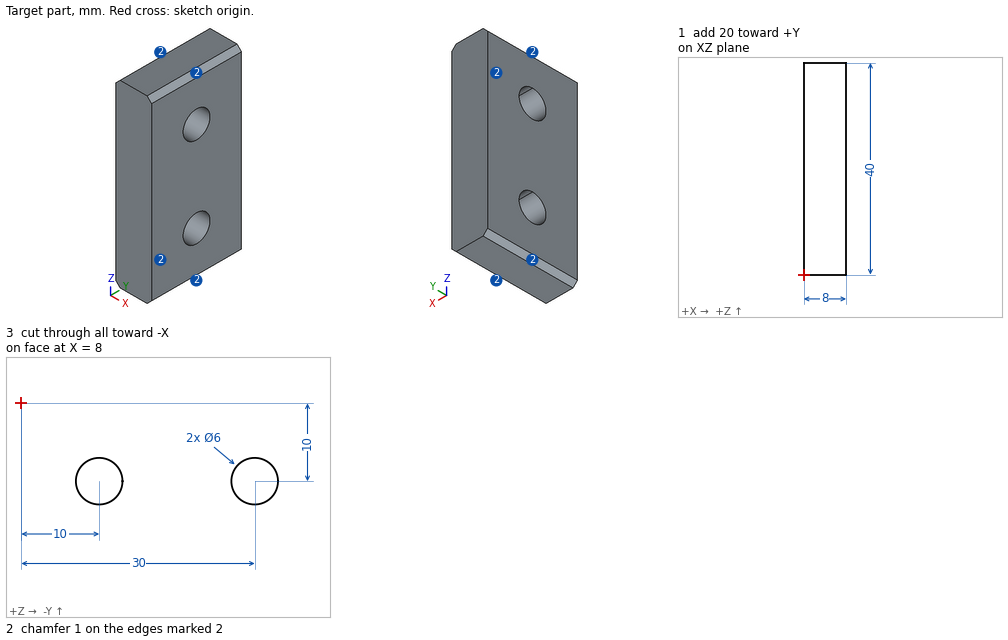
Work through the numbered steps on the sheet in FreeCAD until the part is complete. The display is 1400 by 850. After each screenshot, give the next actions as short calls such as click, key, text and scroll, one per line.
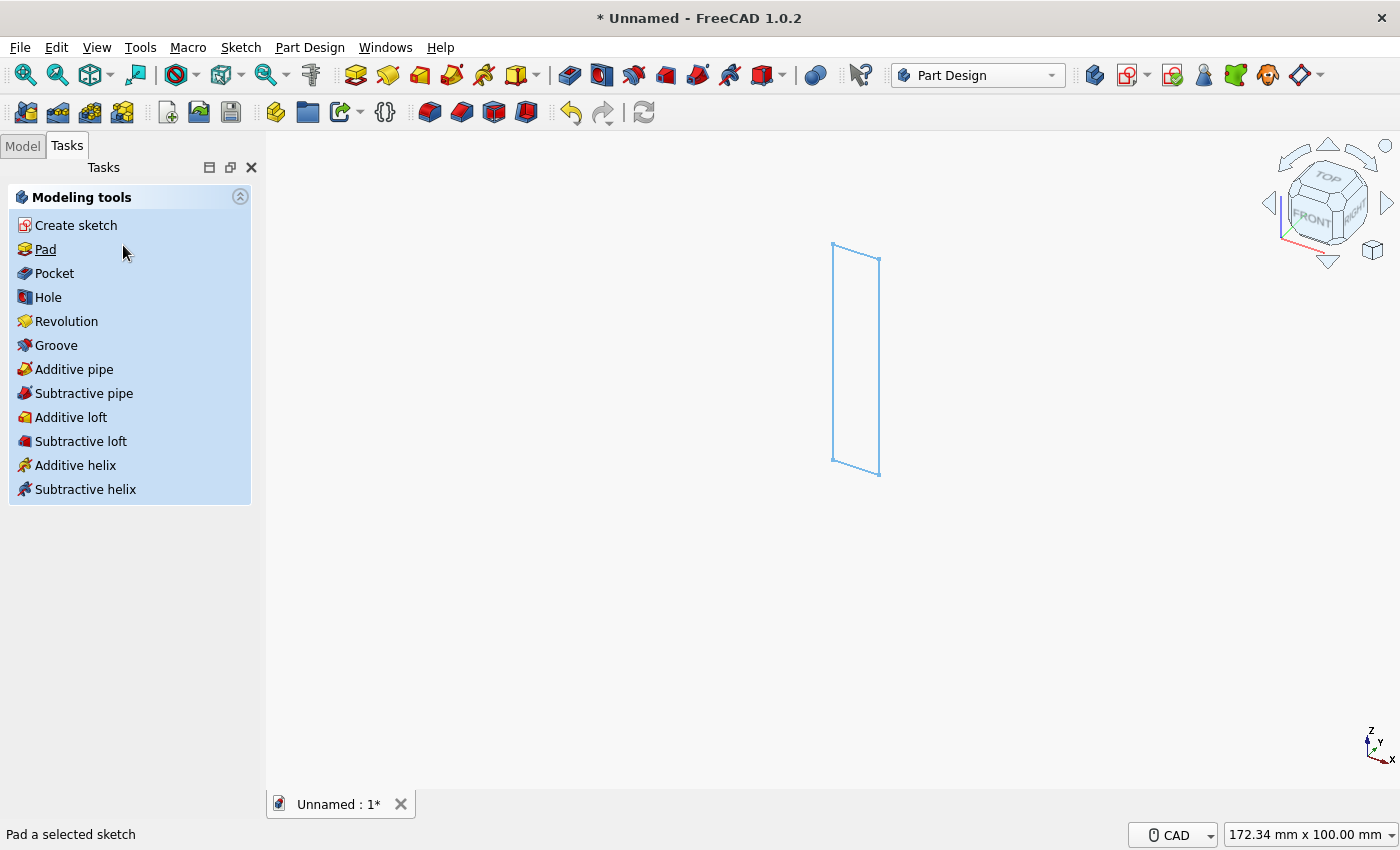
click(356, 76)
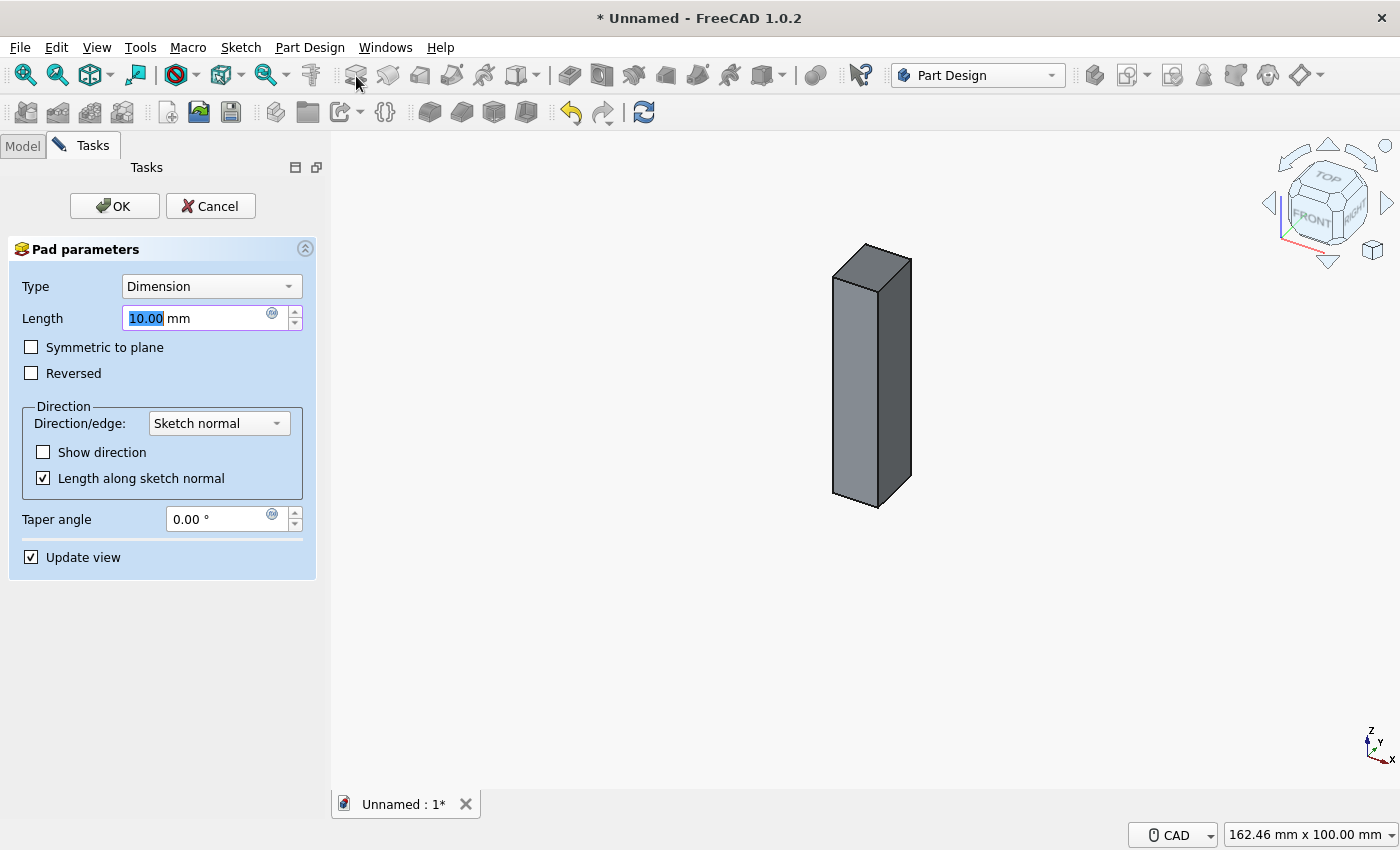
text(20)
key(Tab)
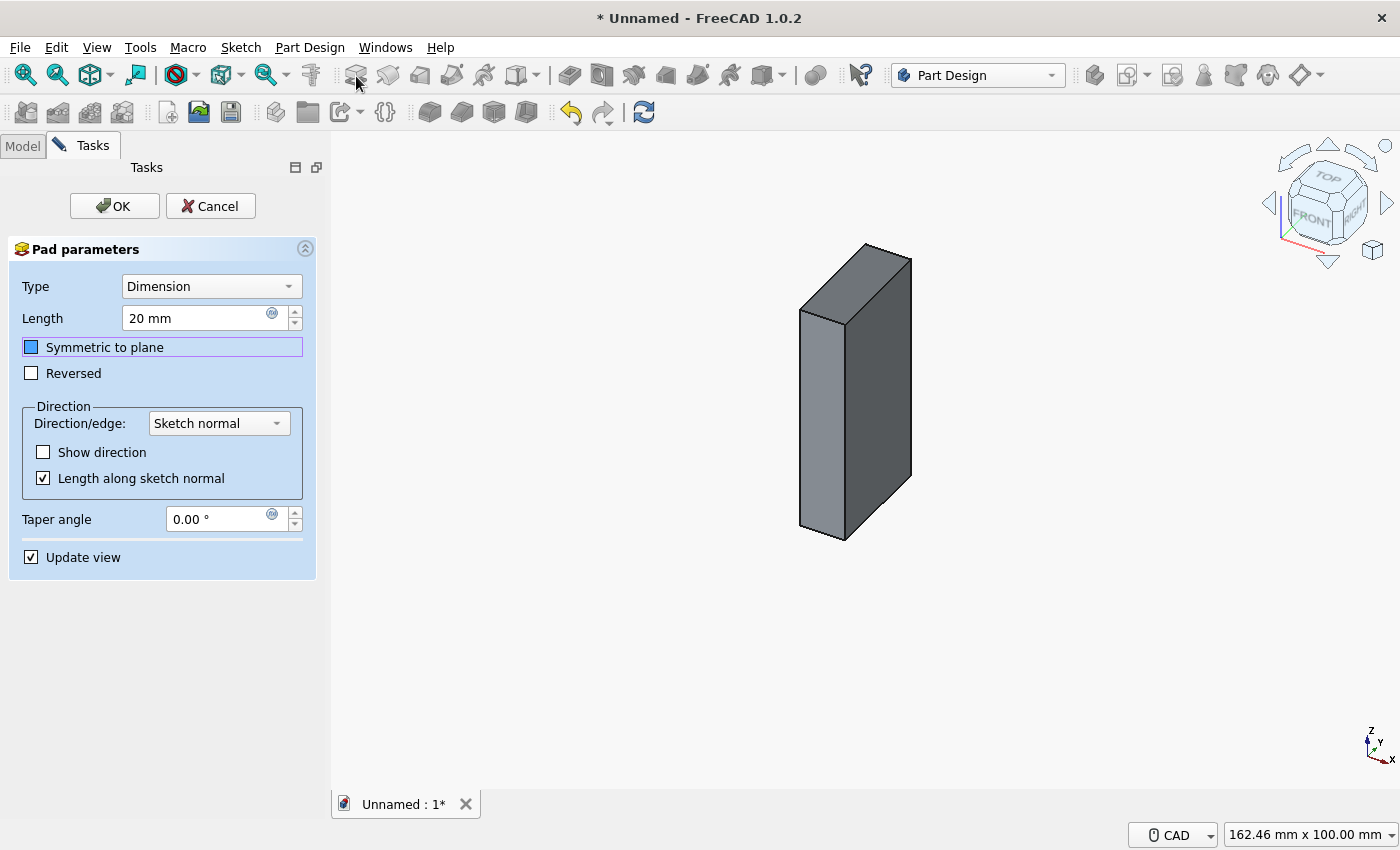
click(30, 373)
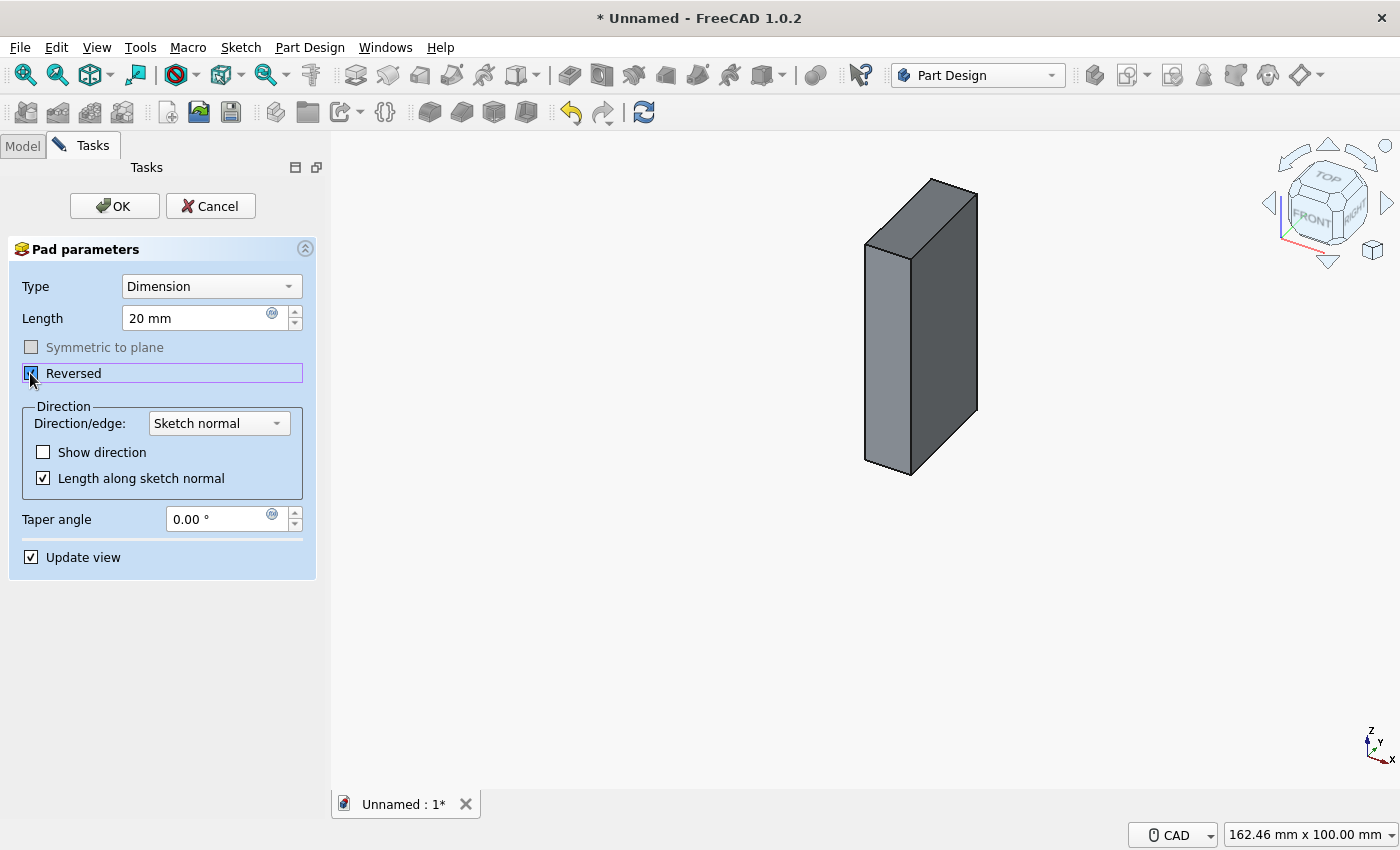
click(115, 206)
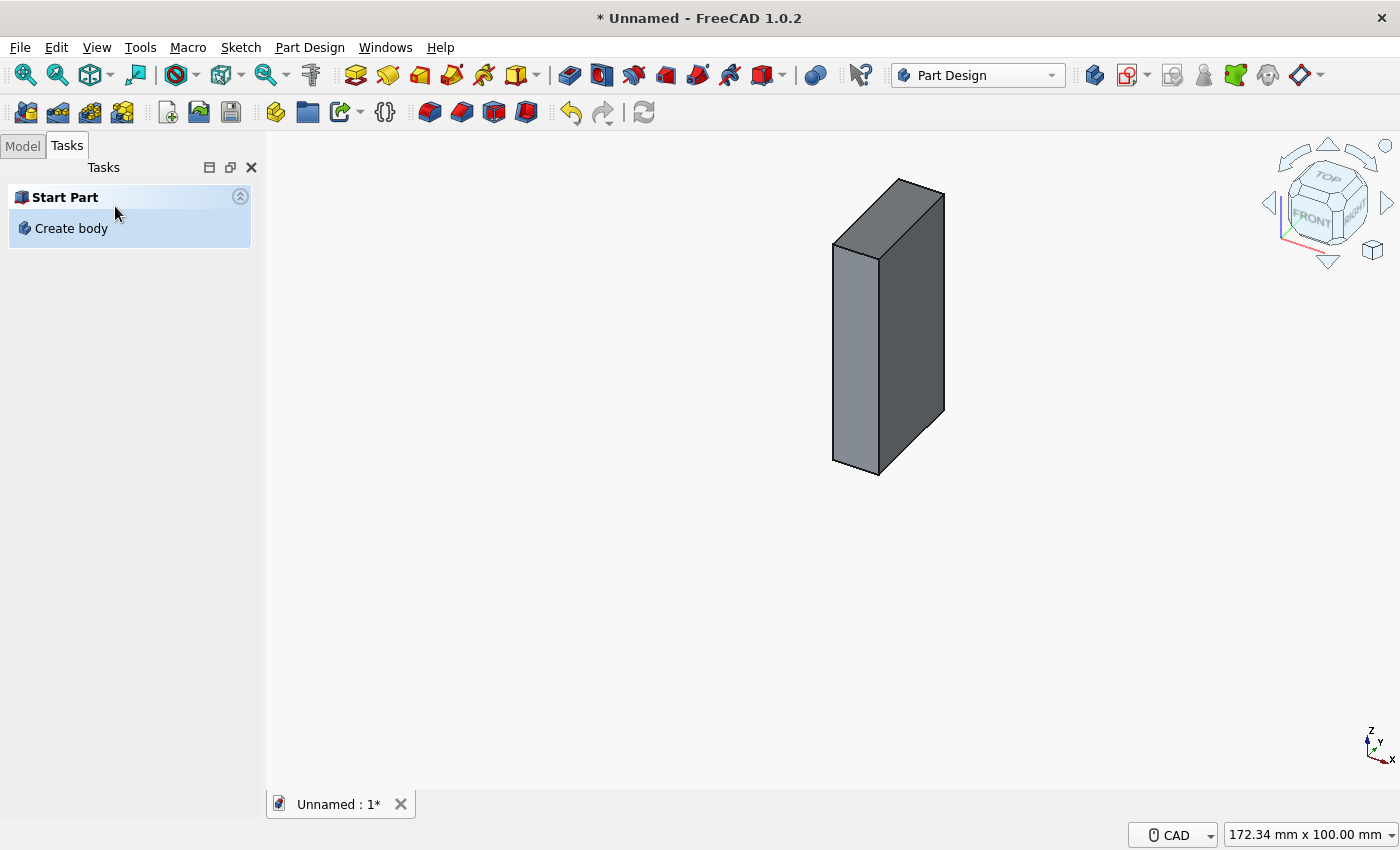
click(26, 76)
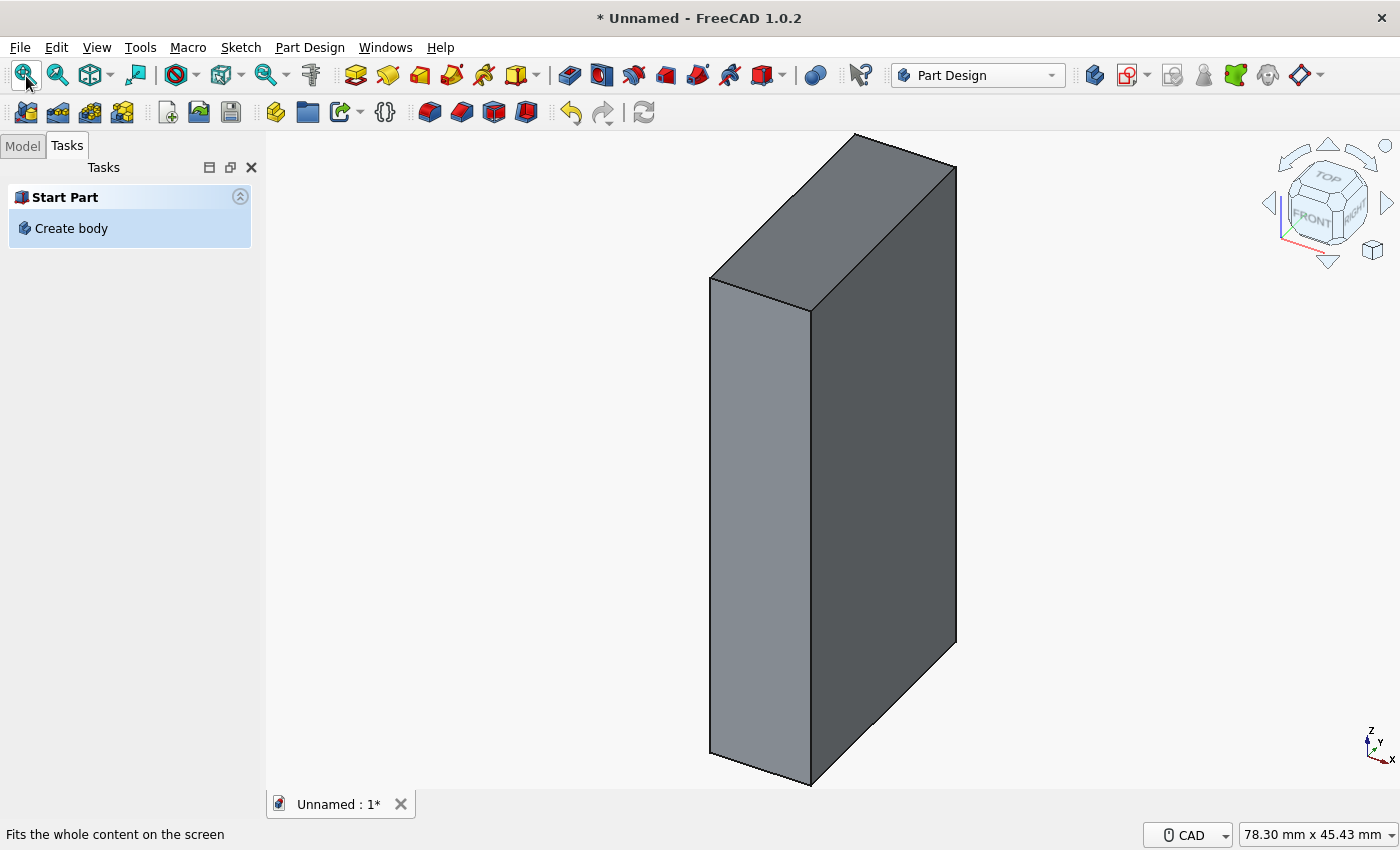
click(883, 238)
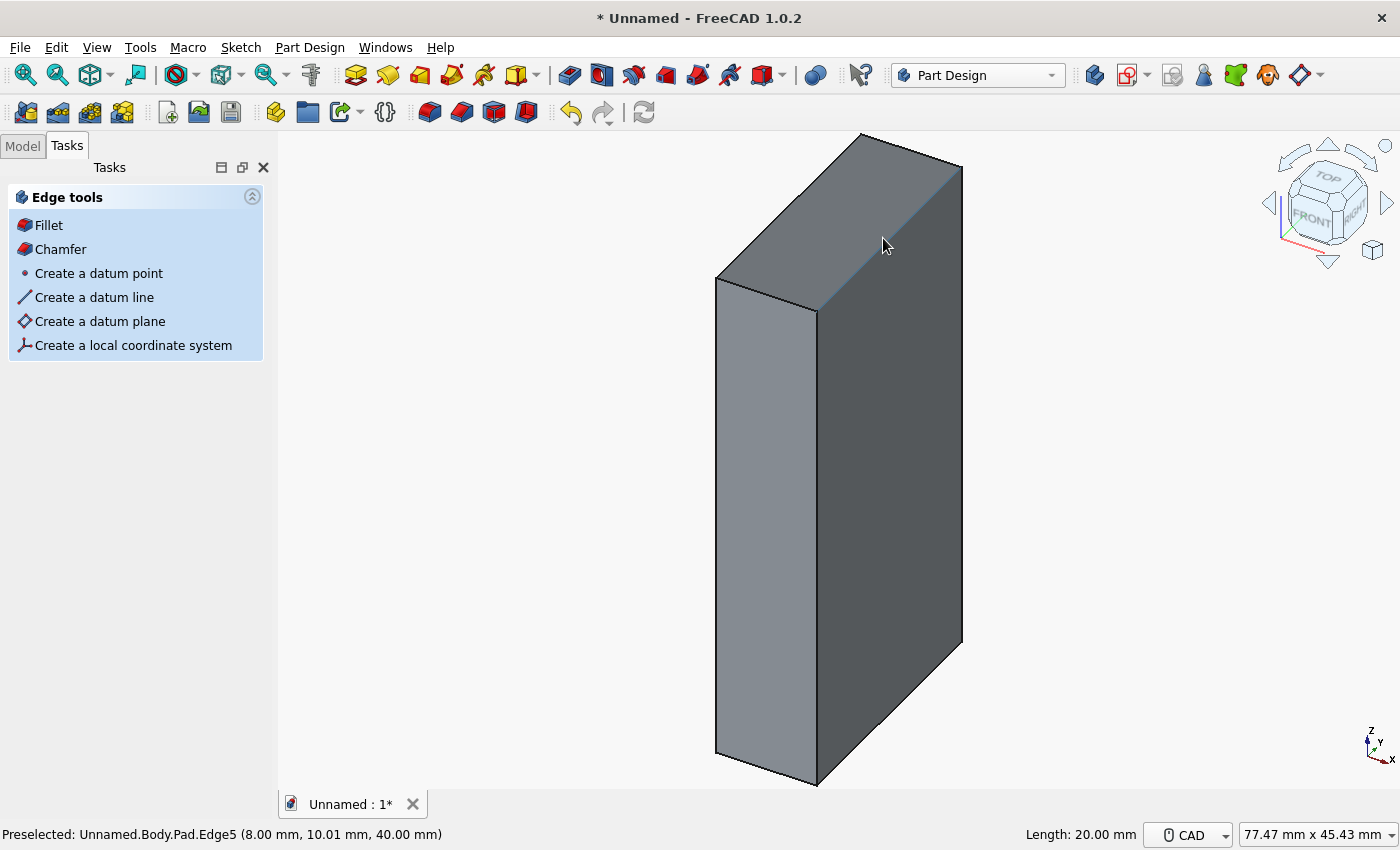
key(0)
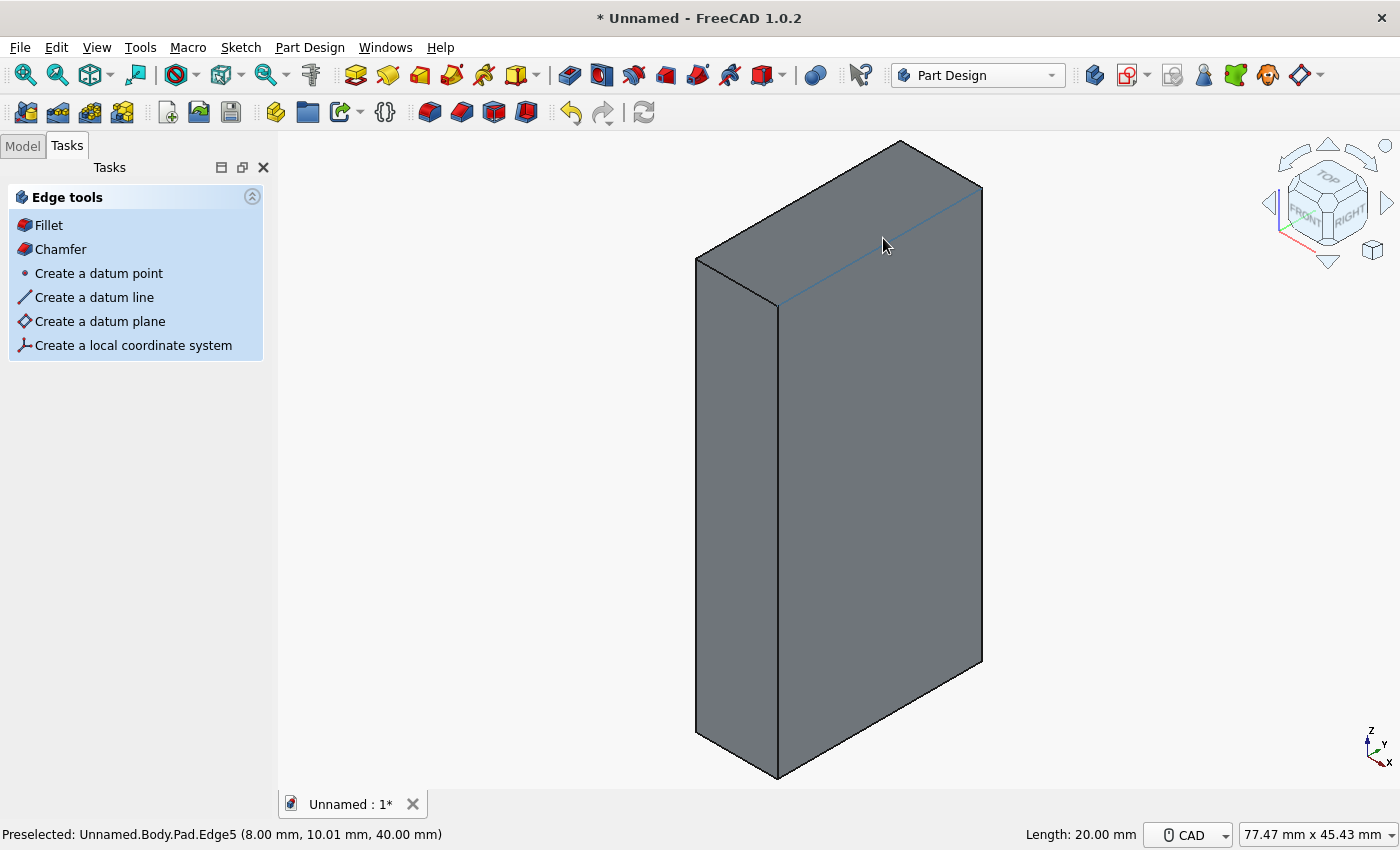
key(2)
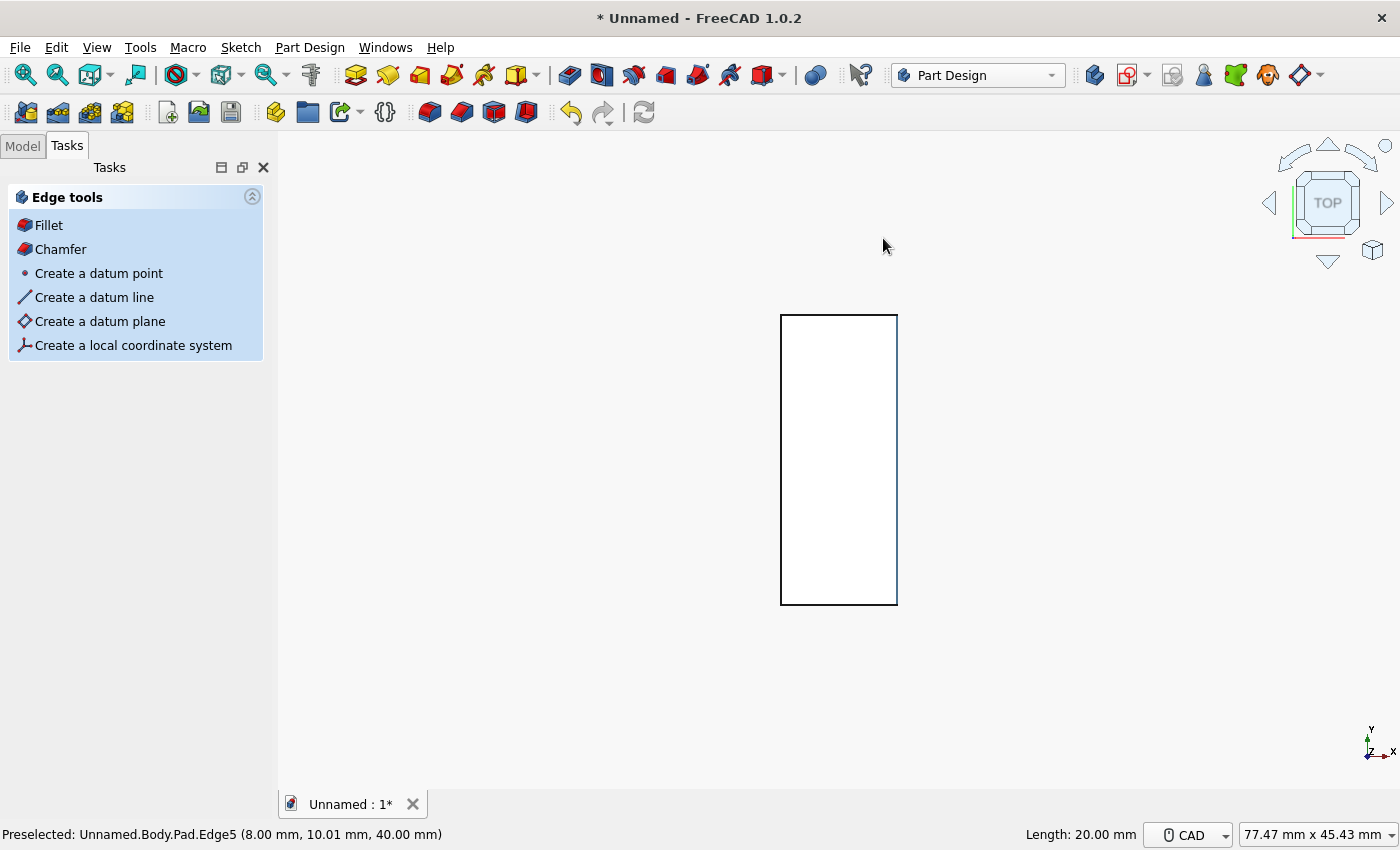
click(26, 76)